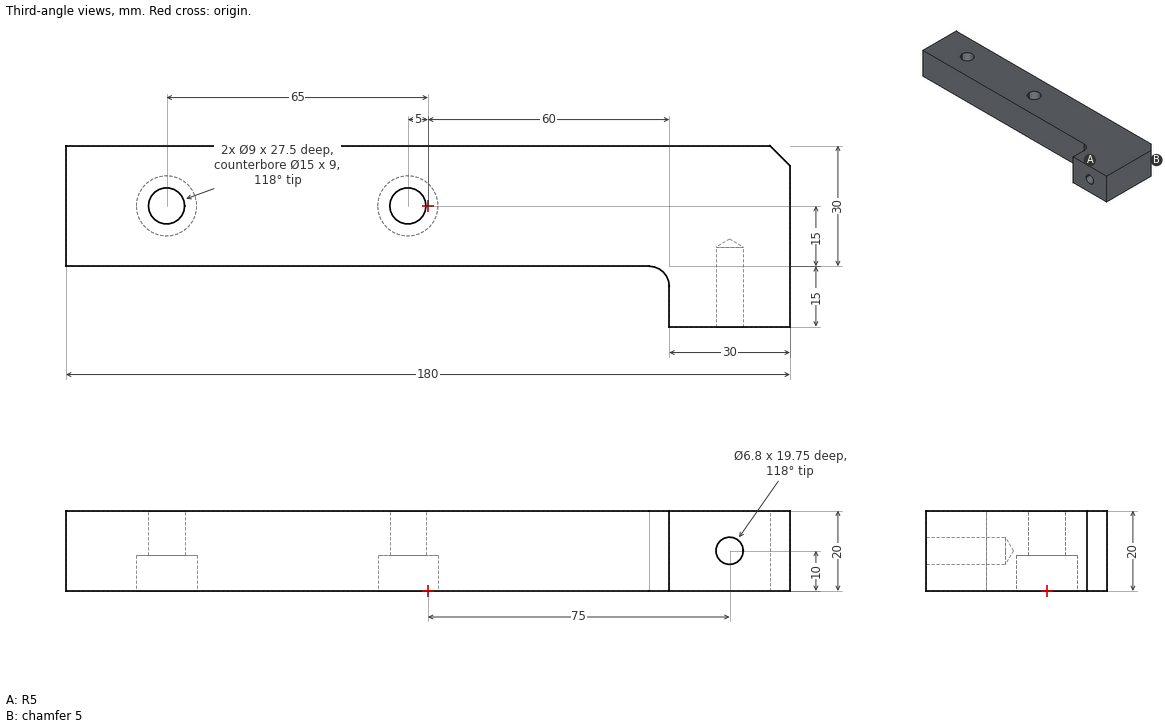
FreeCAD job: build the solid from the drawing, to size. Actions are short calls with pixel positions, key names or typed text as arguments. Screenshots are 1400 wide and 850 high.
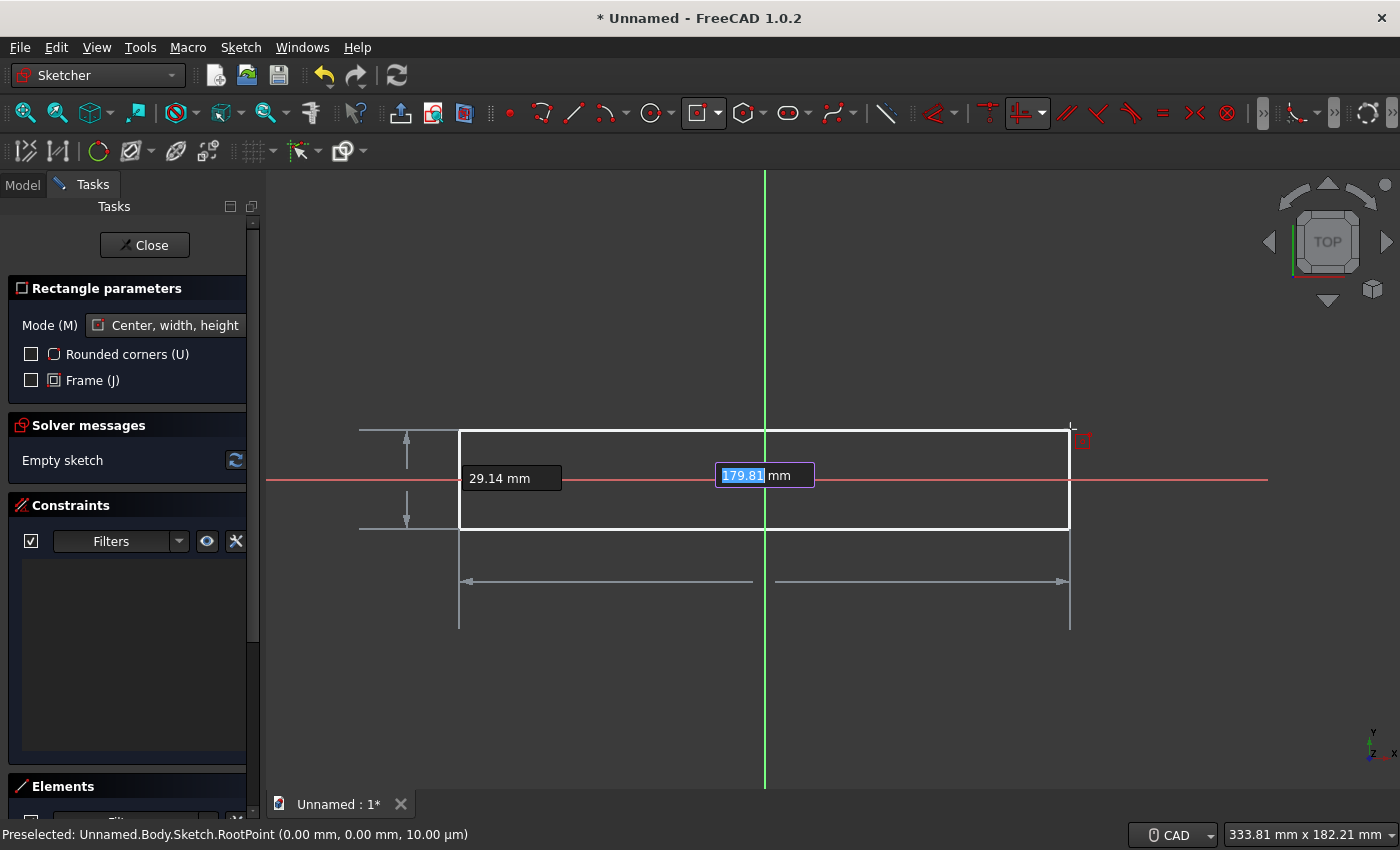
text(180)
key(Tab)
text(30)
key(Return)
key(Escape)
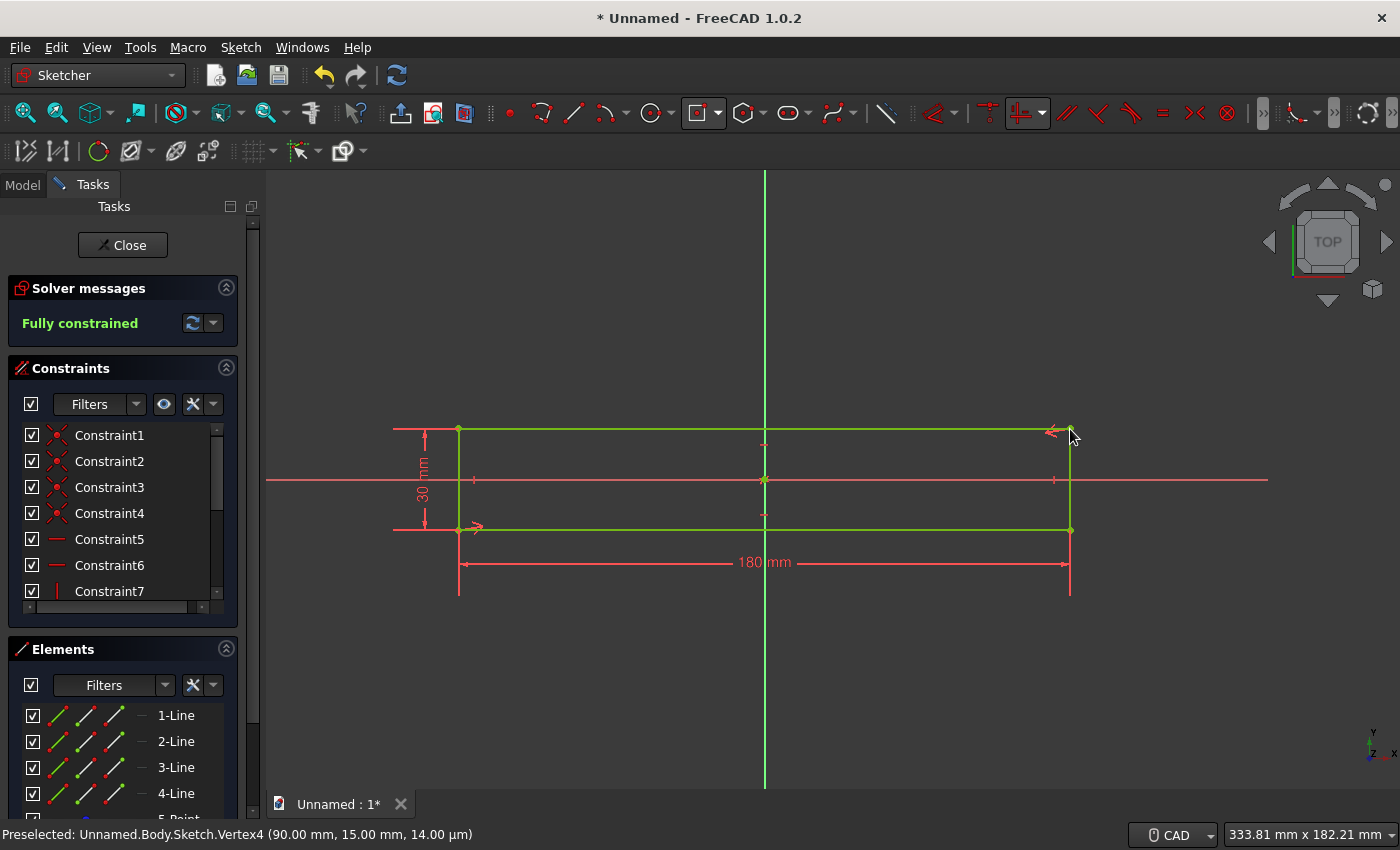
click(123, 245)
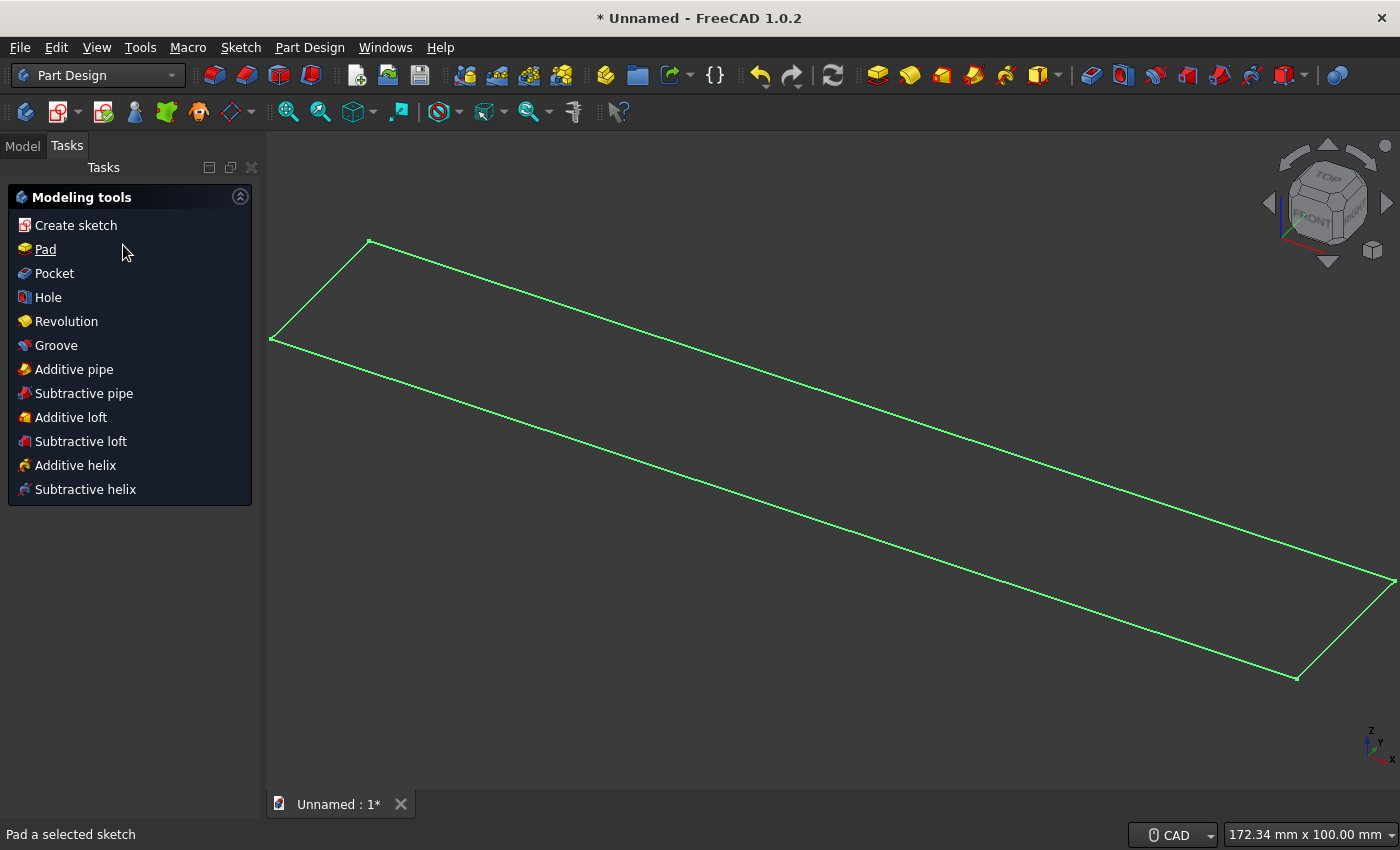
click(878, 76)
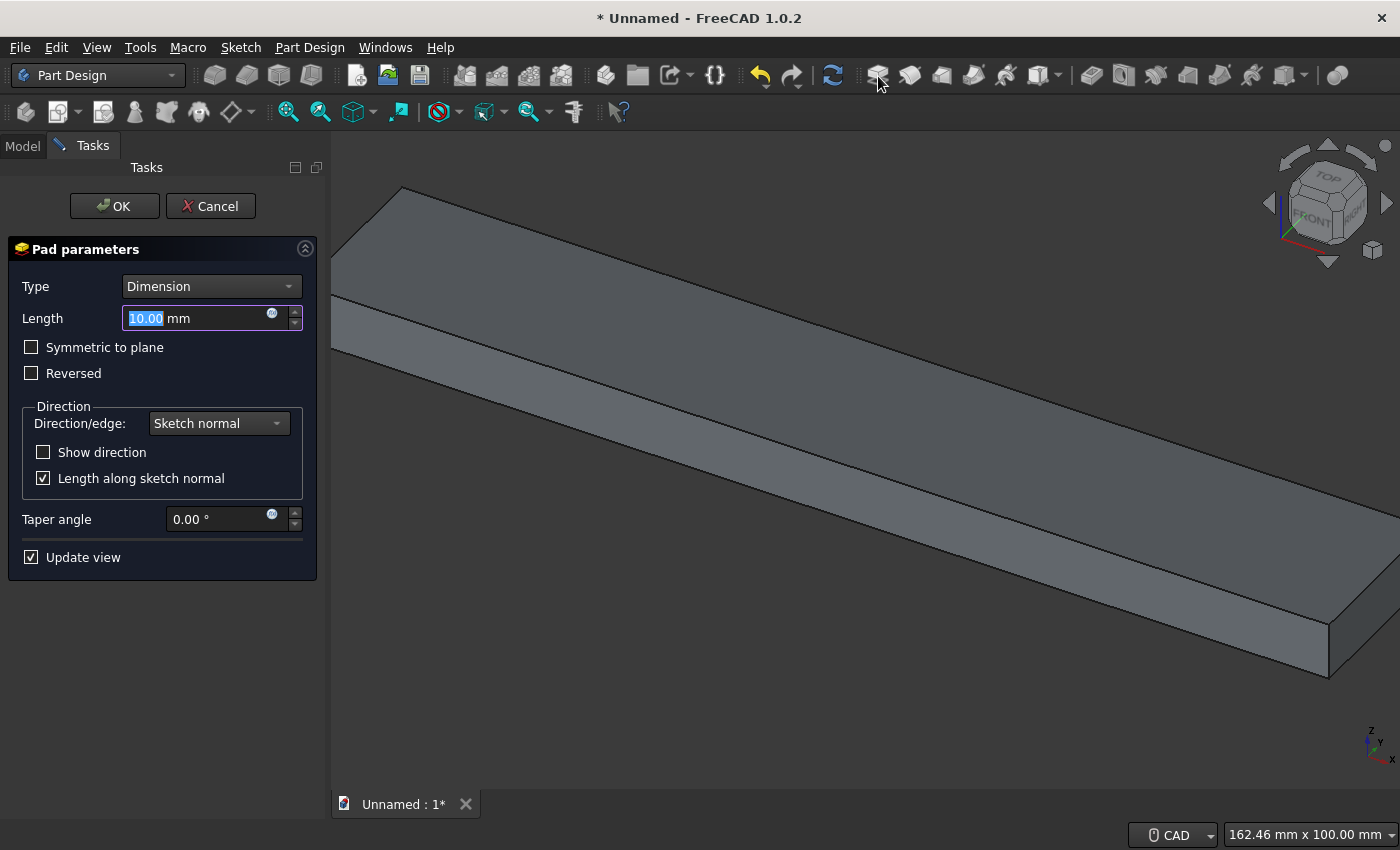
text(20)
key(Tab)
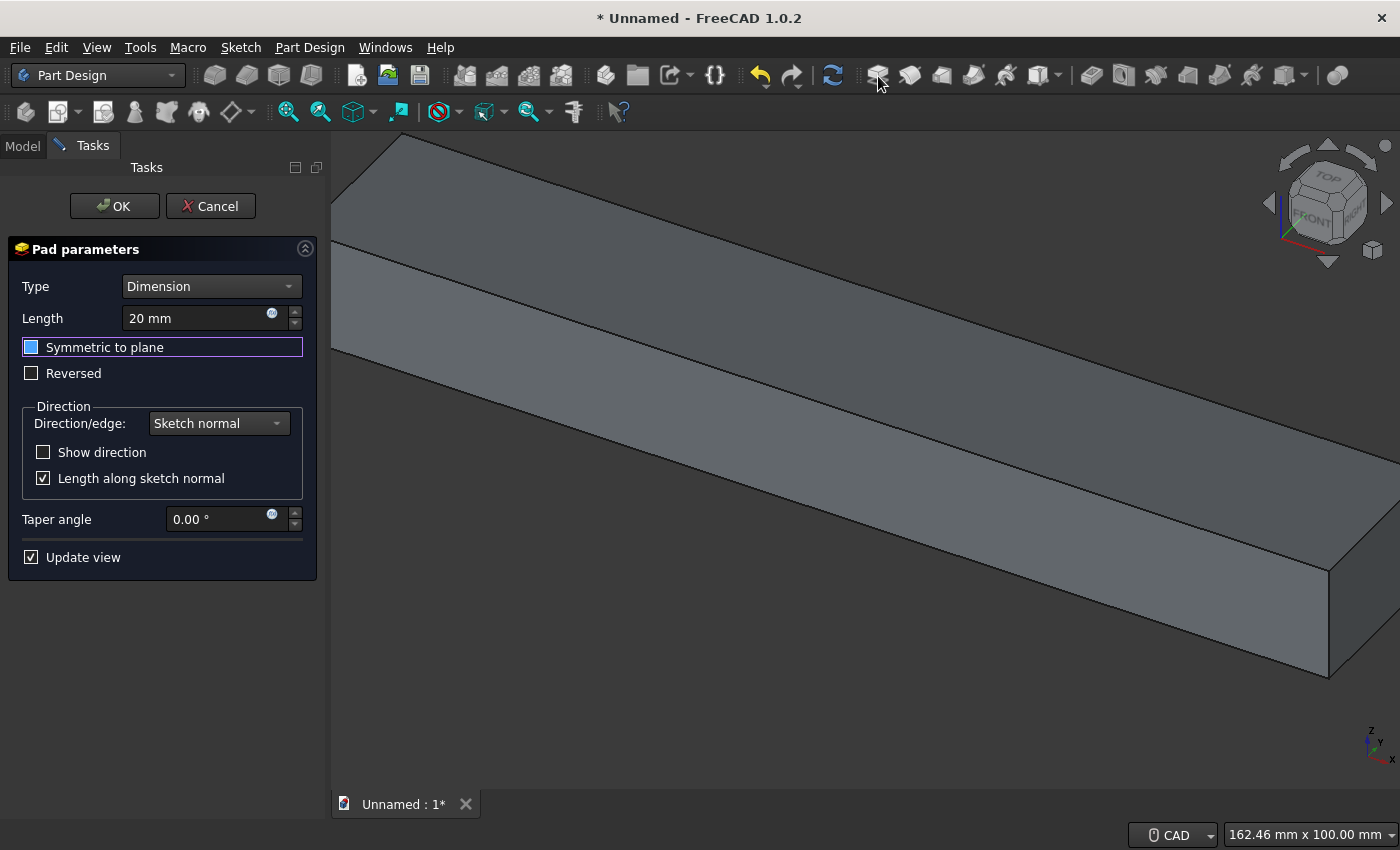
click(115, 206)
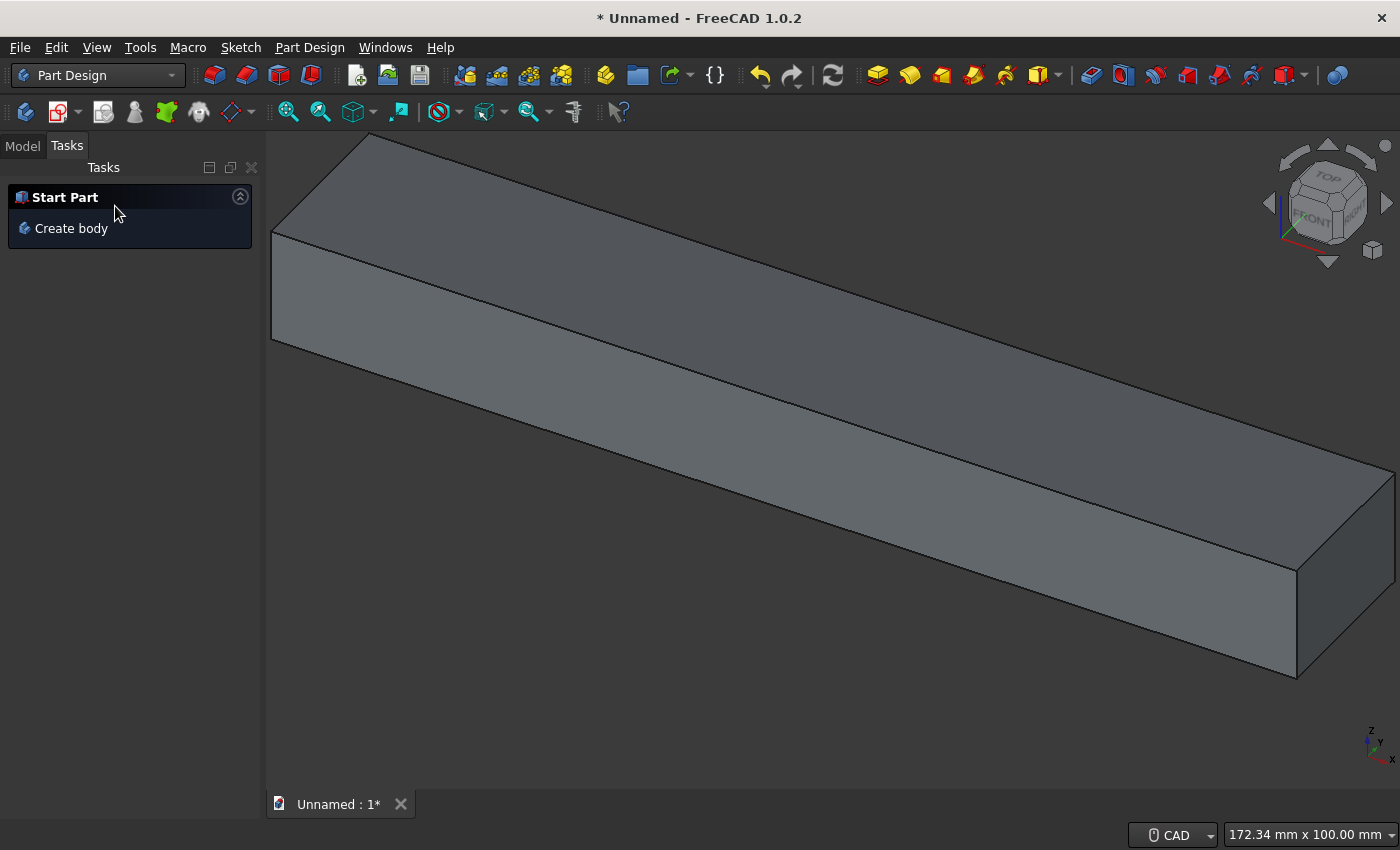
click(1126, 448)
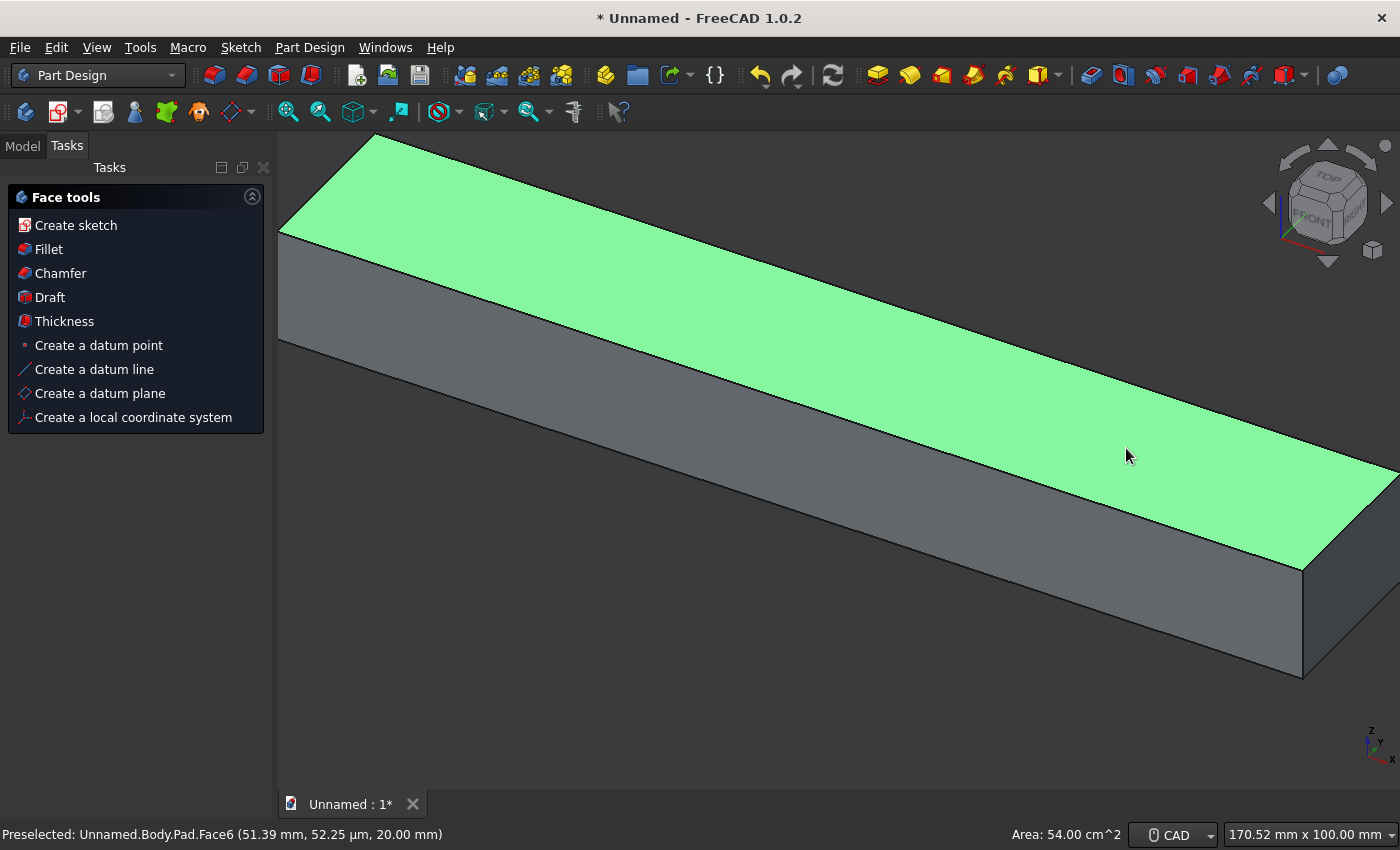
click(58, 112)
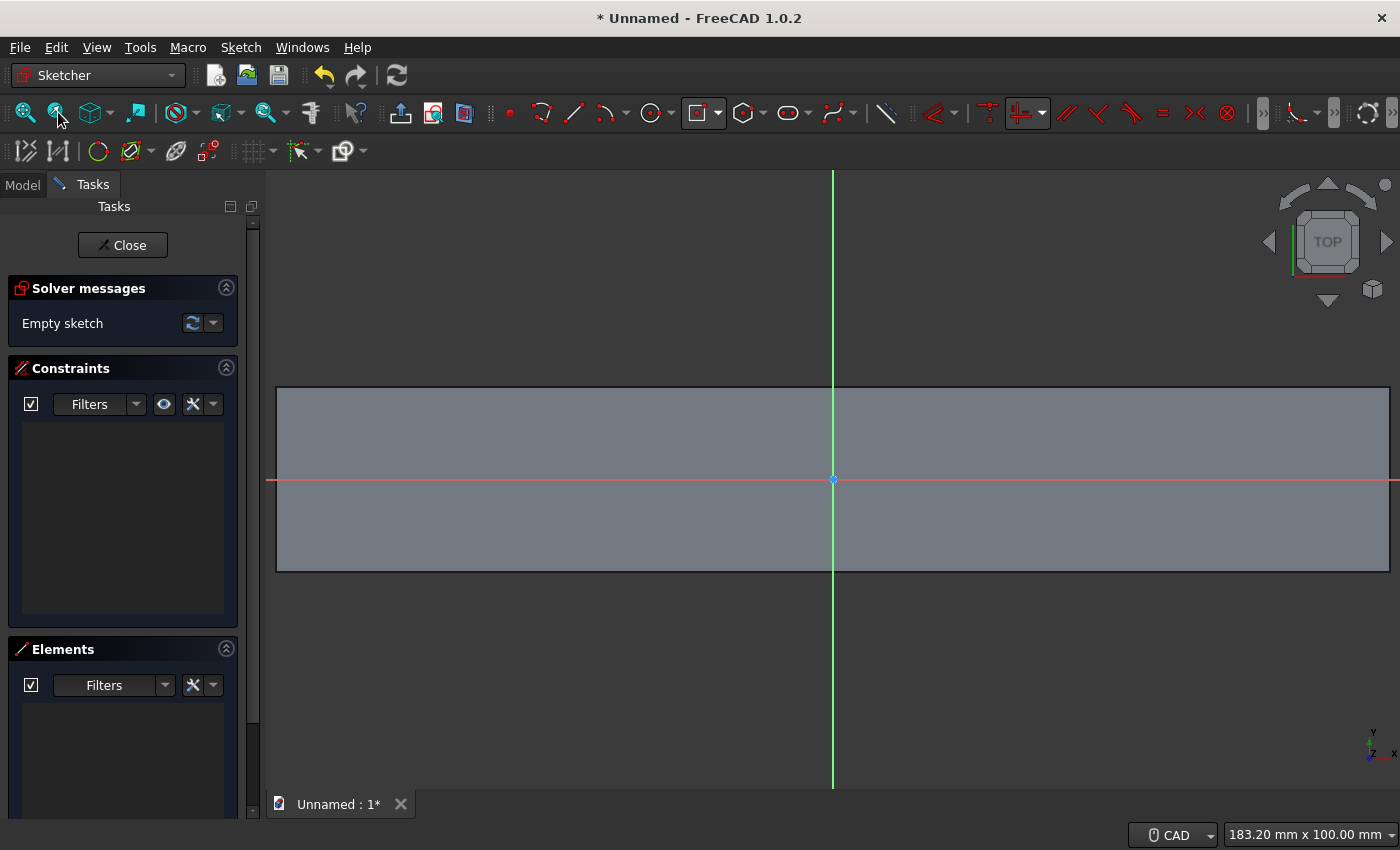
scroll(764, 480, down, 5)